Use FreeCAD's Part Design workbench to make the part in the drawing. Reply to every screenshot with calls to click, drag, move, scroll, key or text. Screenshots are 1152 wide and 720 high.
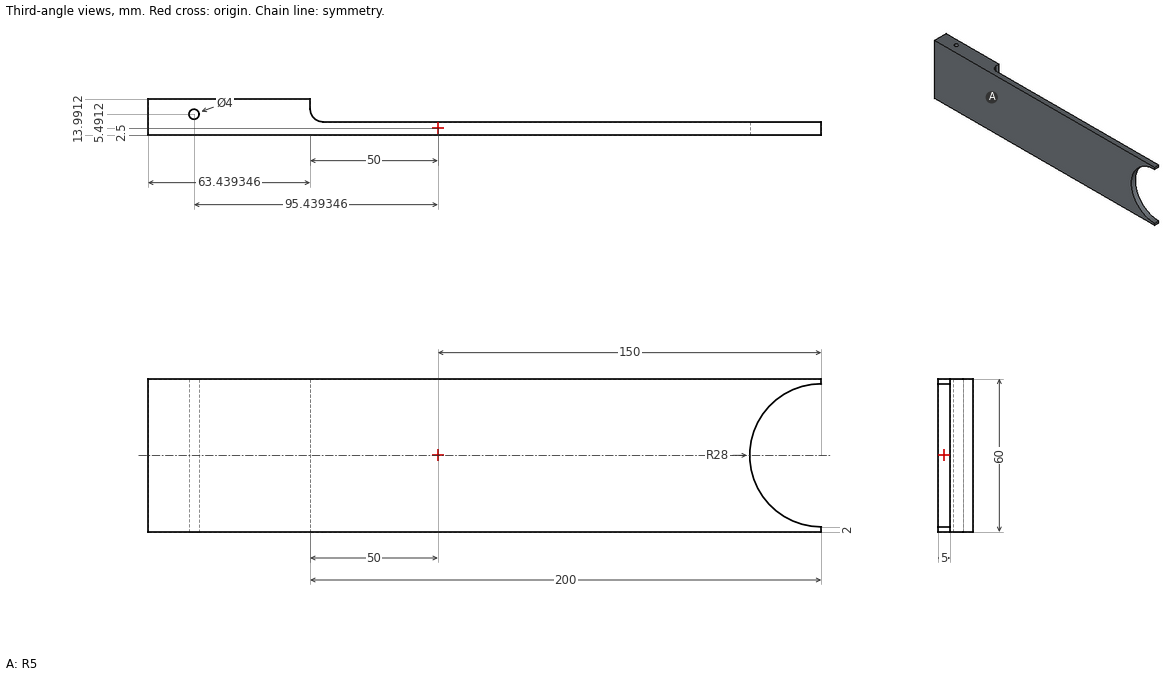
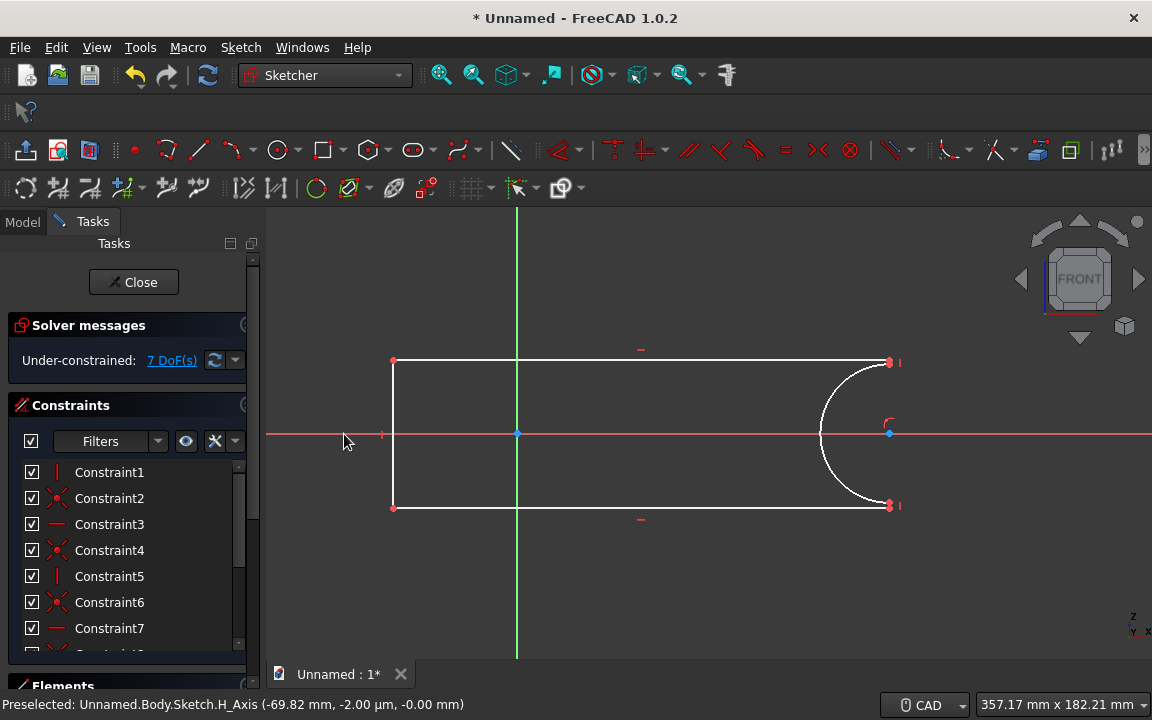
scroll(889, 508, up, 5)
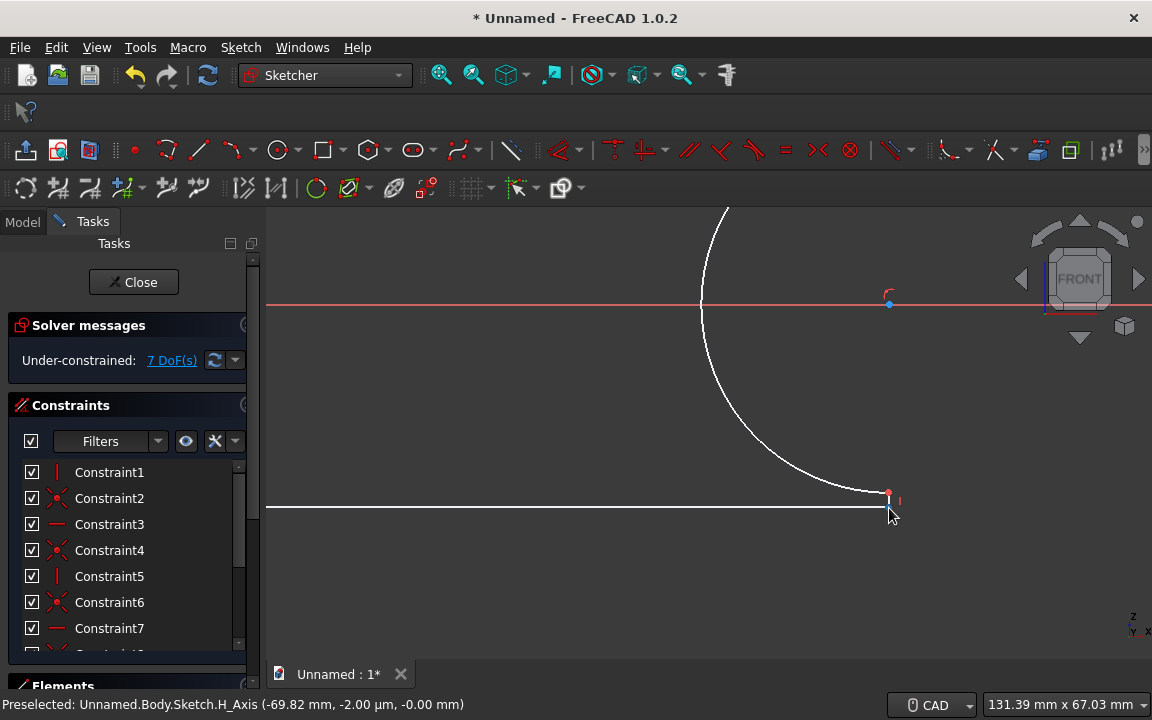
click(889, 507)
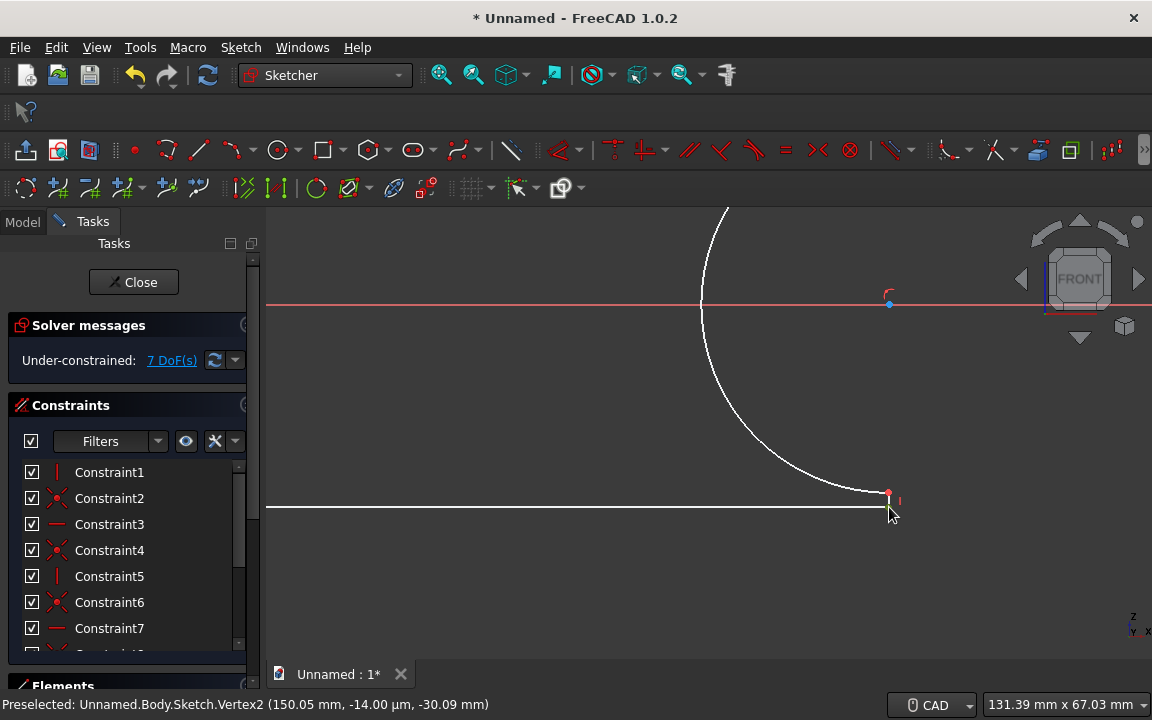
scroll(889, 508, down, 5)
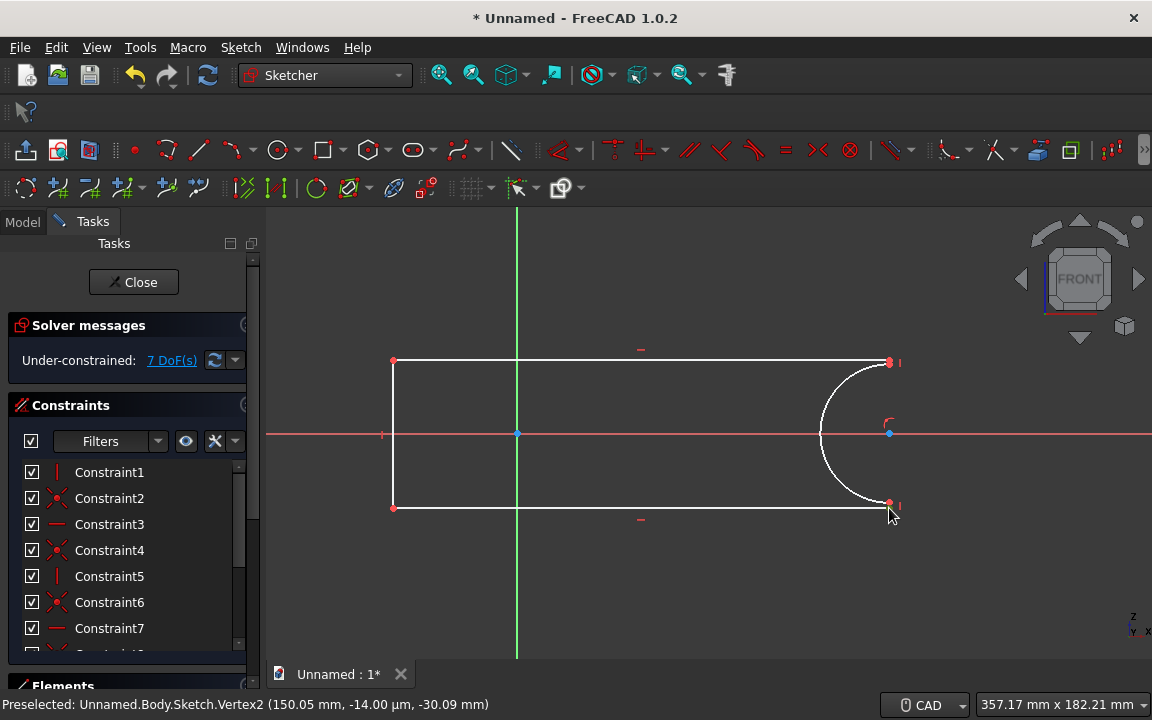
scroll(889, 360, up, 6)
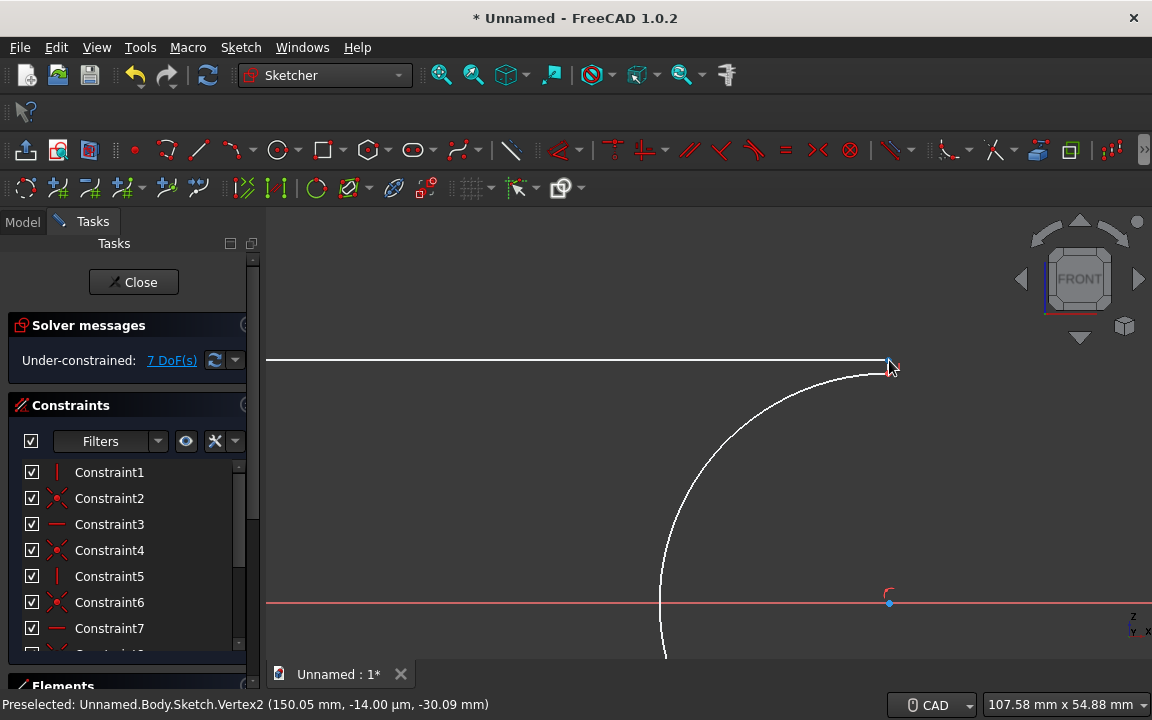
click(888, 360)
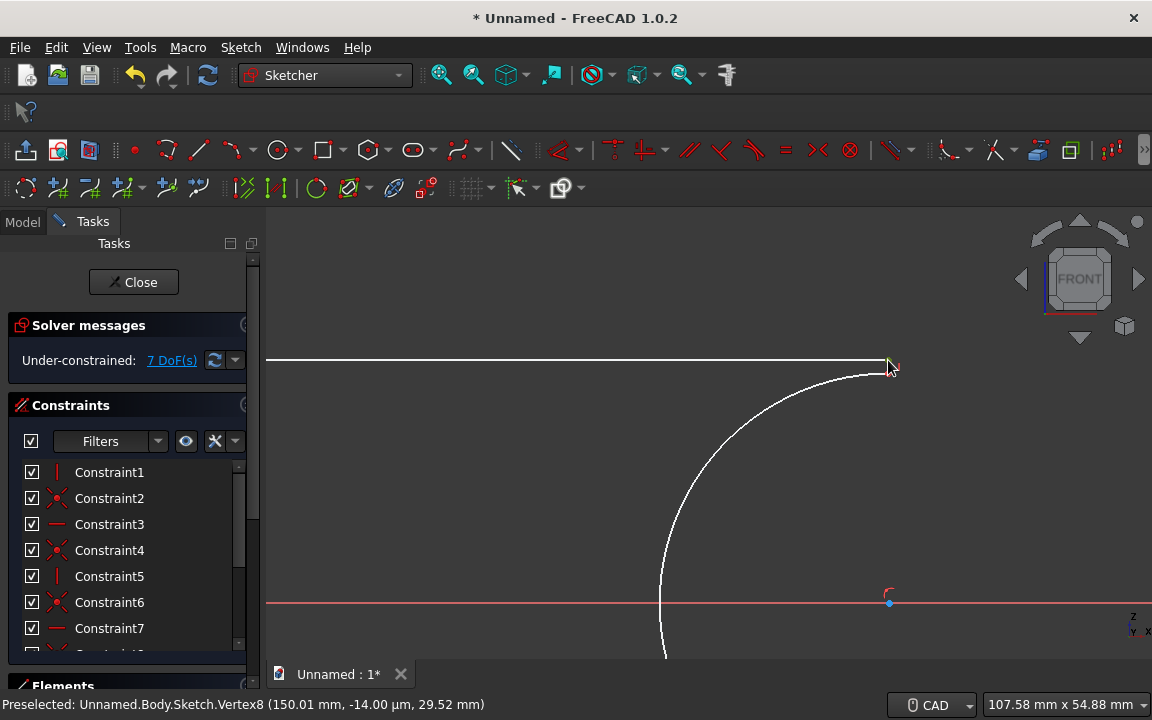
click(344, 603)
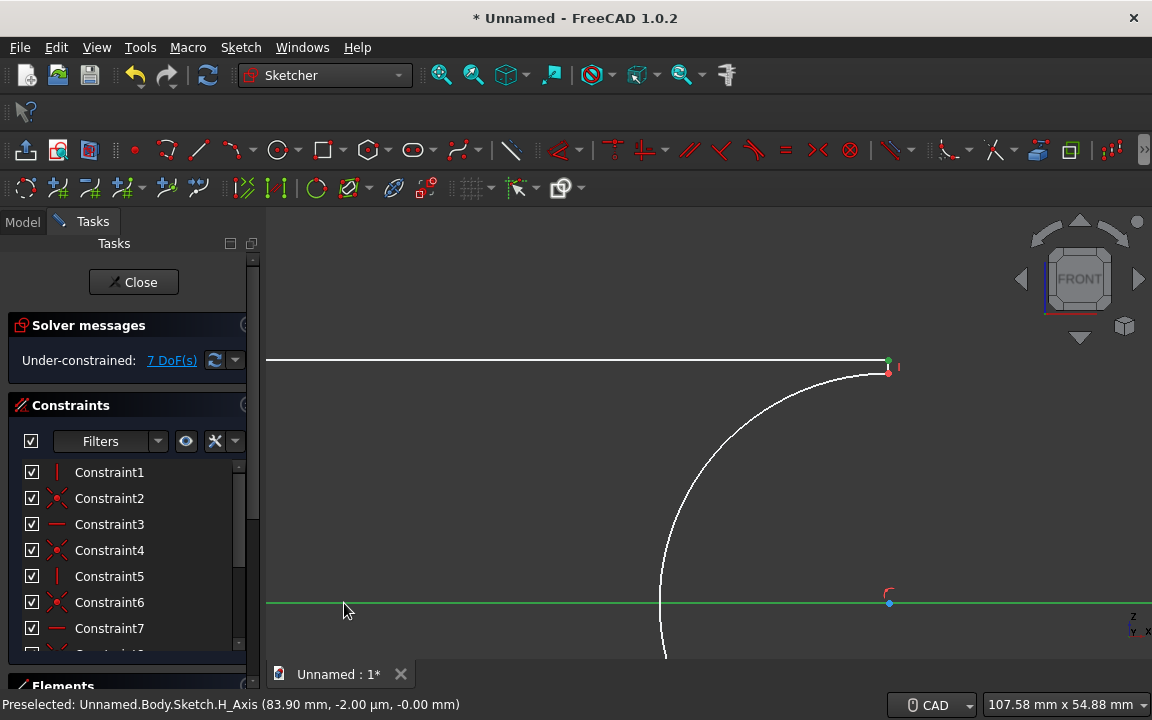
click(818, 150)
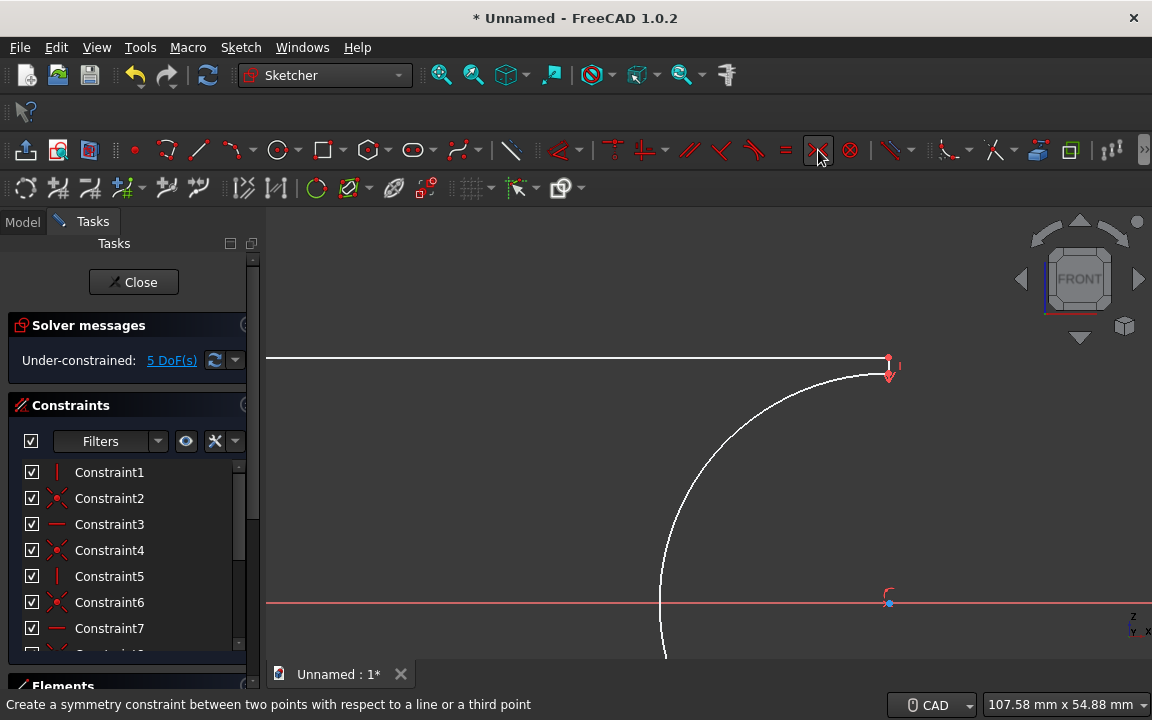
click(558, 150)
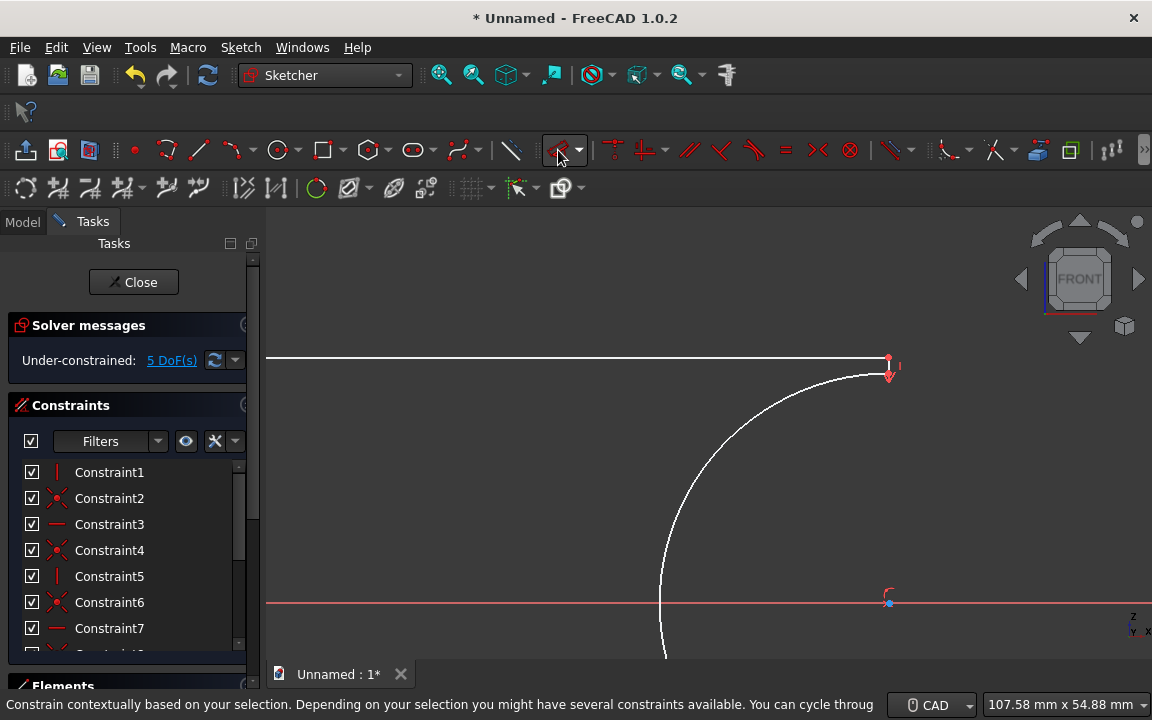
click(703, 469)
click(677, 450)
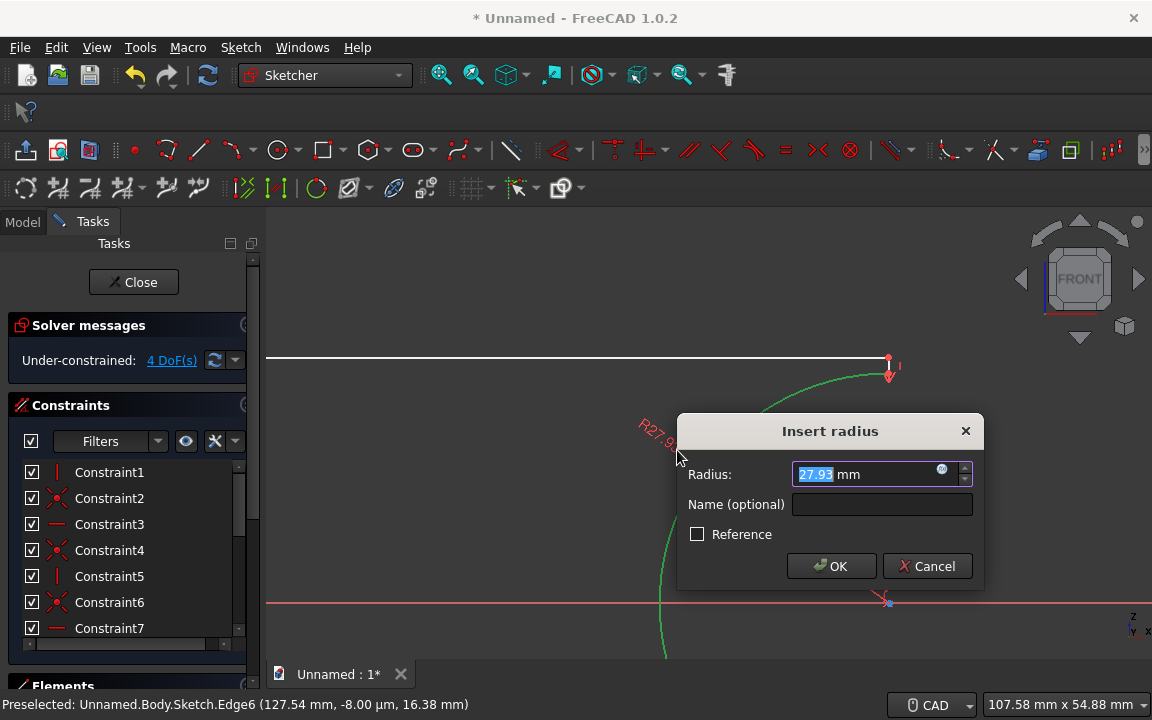
text(28)
key(Return)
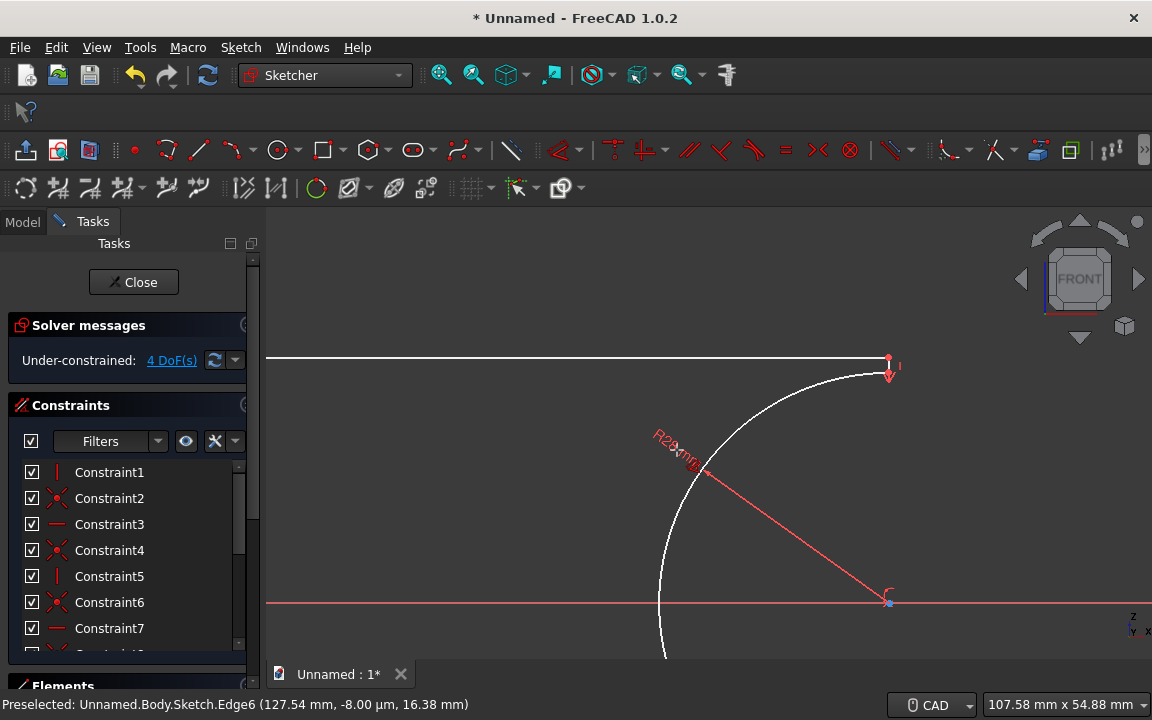
scroll(889, 360, down, 6)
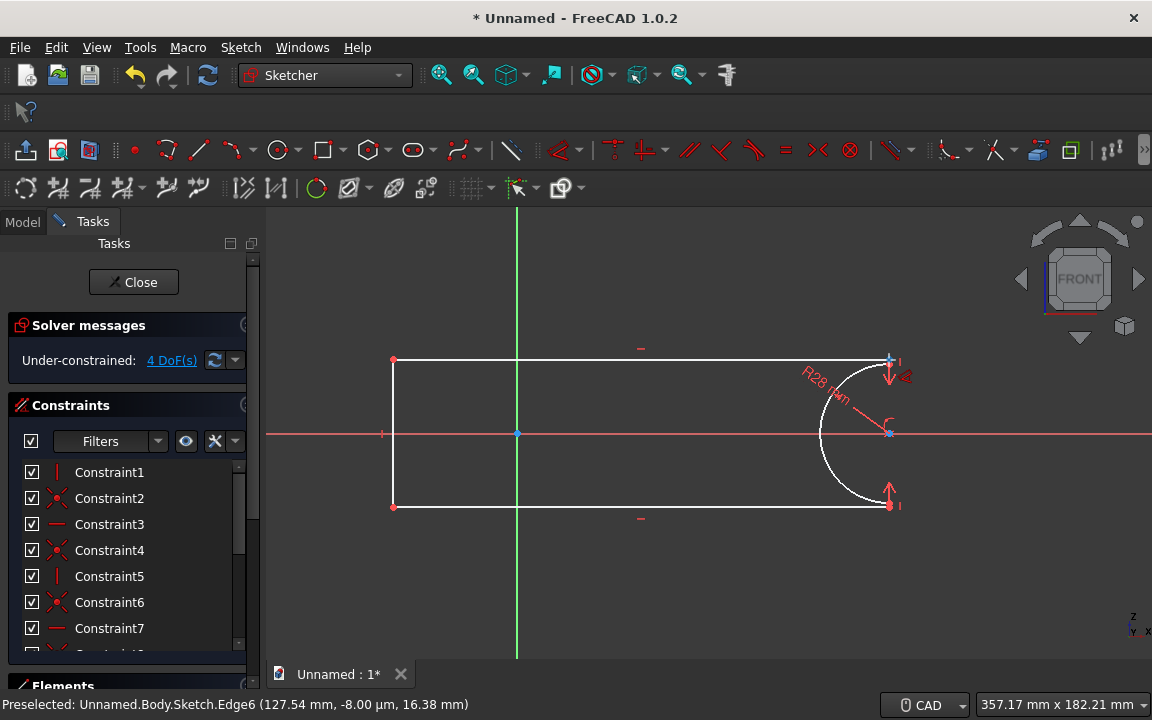
scroll(889, 505, up, 11)